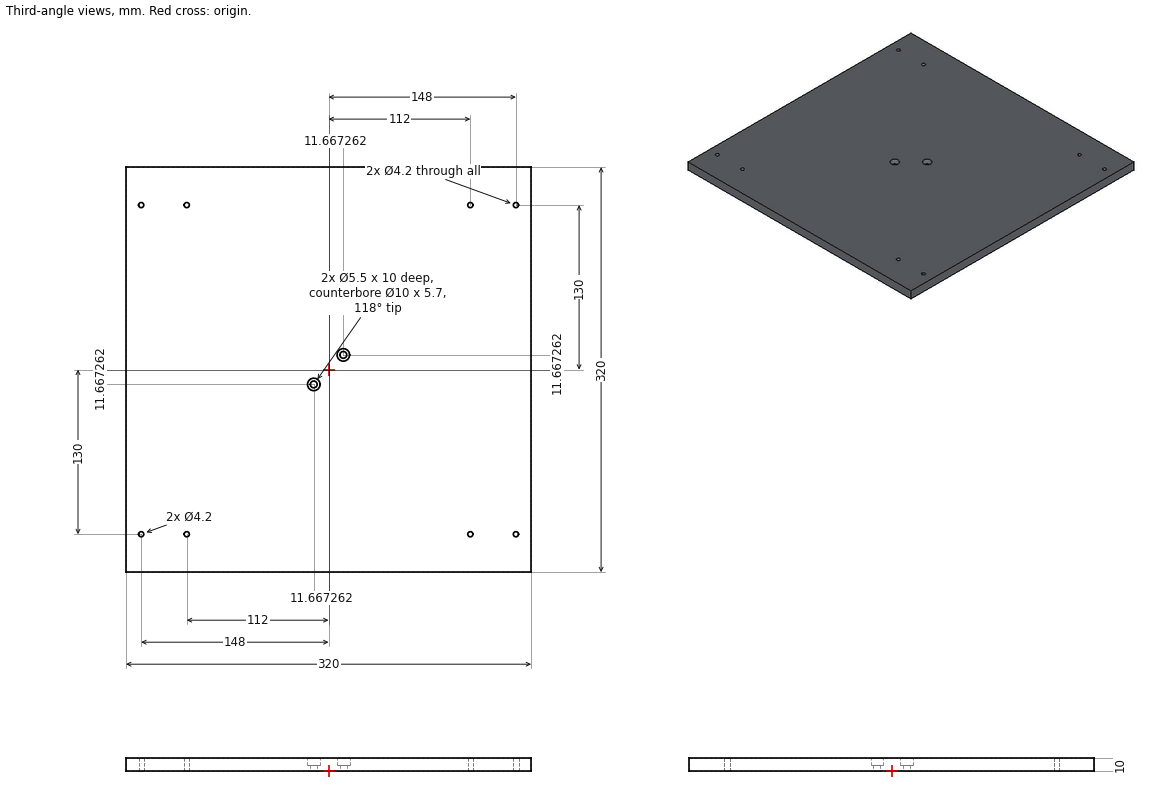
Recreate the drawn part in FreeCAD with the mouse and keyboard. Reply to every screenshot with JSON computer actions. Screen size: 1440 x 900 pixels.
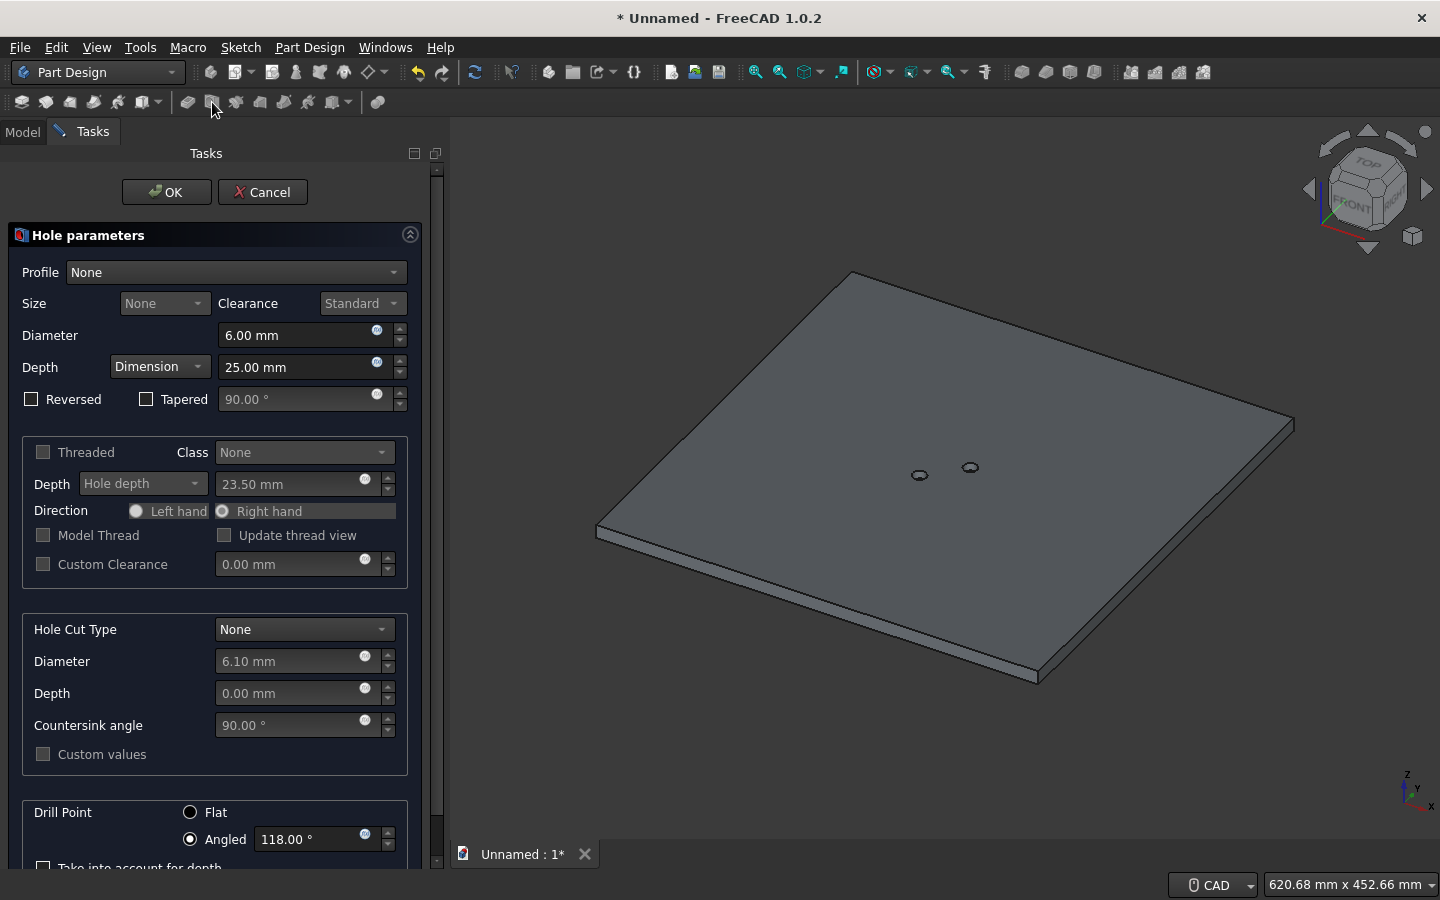
{"action": "triple_click", "coordinate": [305, 335]}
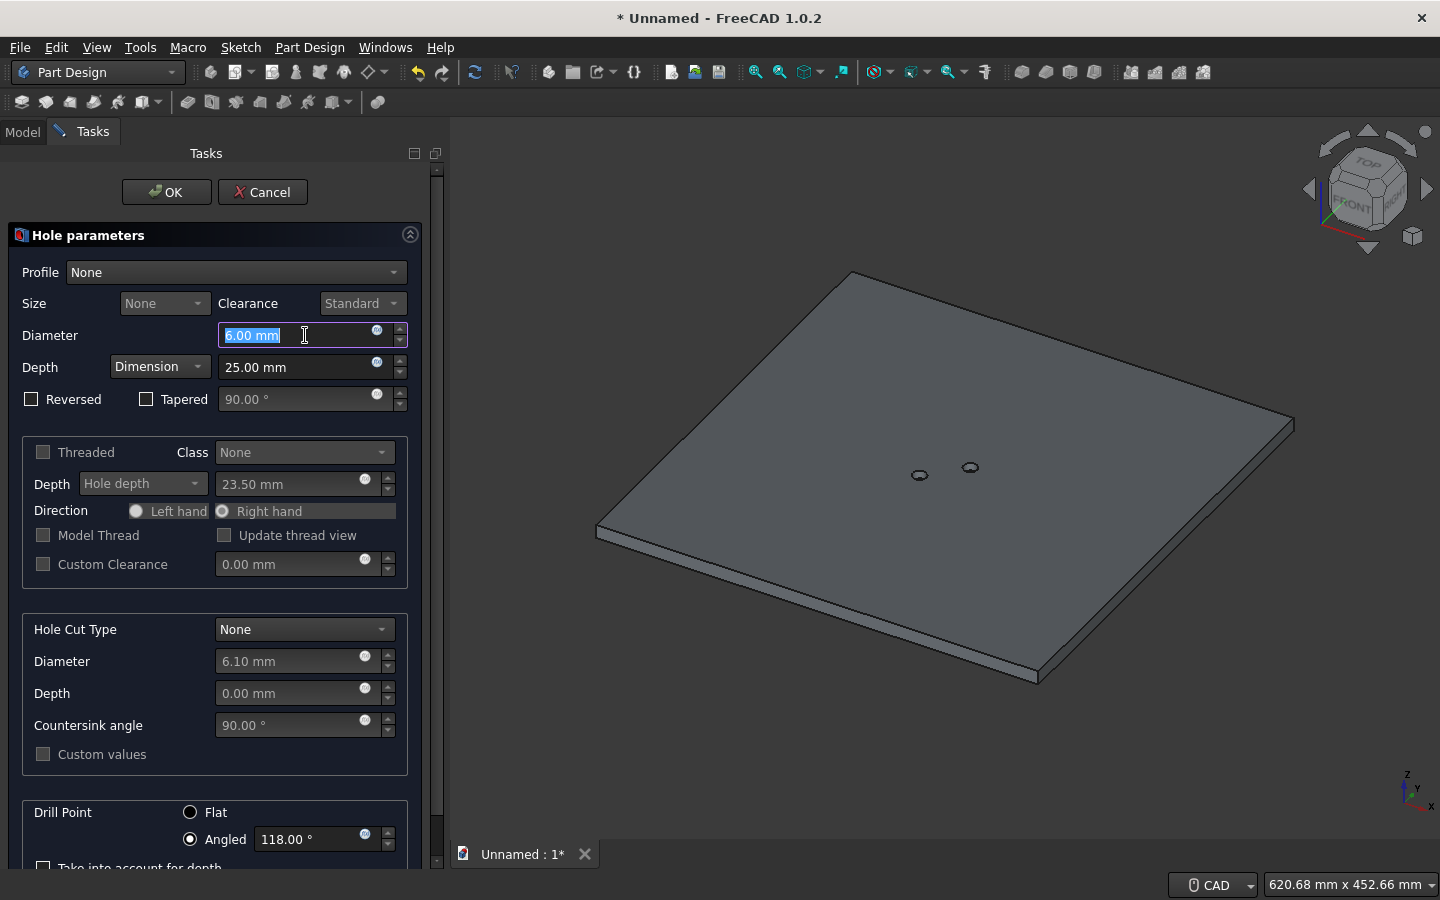
{"action": "type", "text": "4.2"}
{"action": "key", "text": "Tab"}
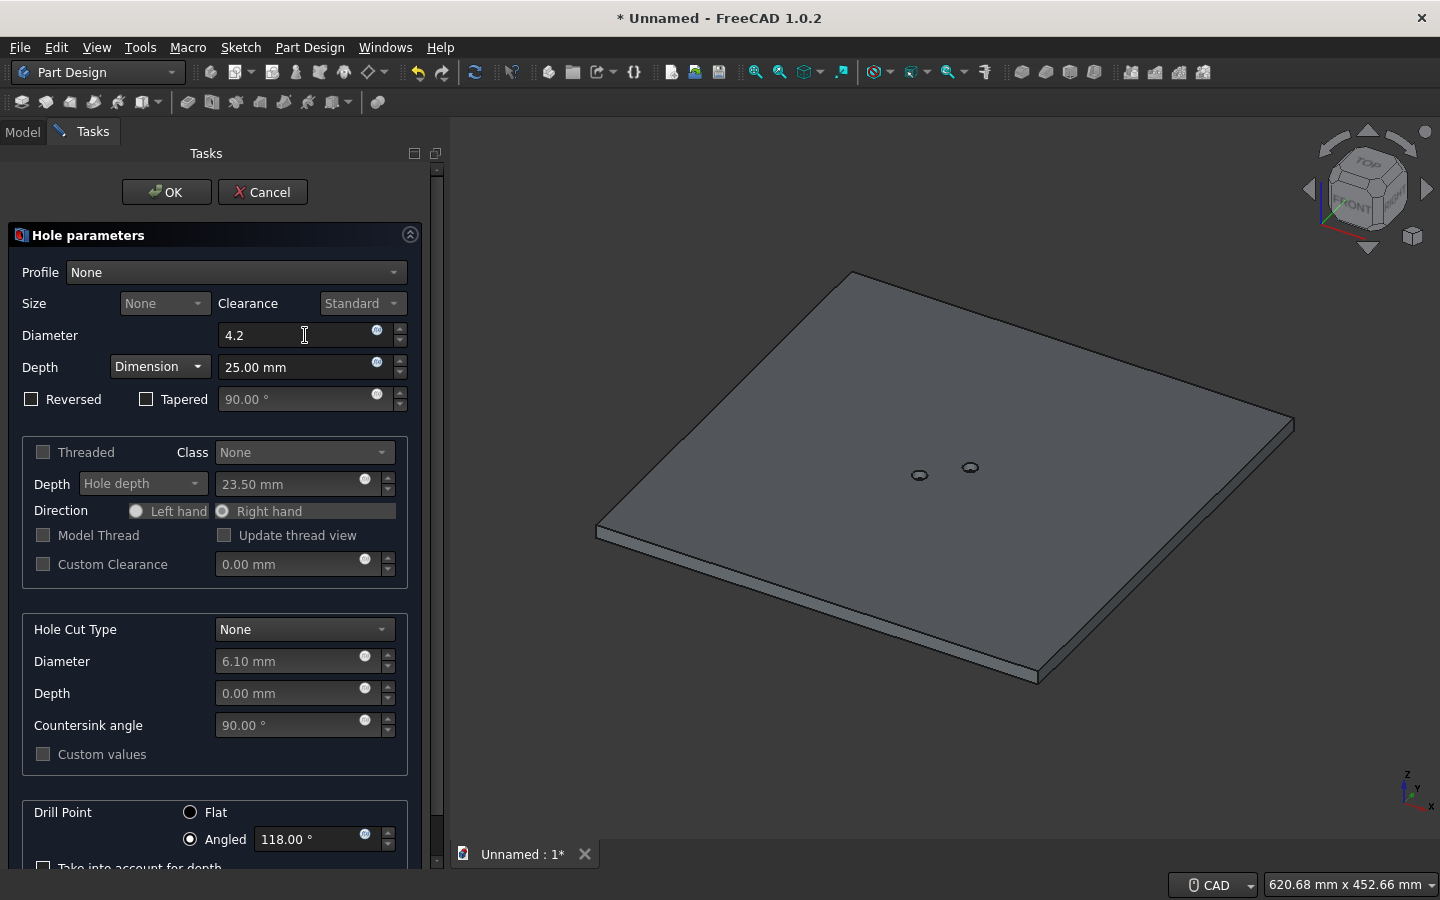
{"action": "left_click", "coordinate": [161, 366]}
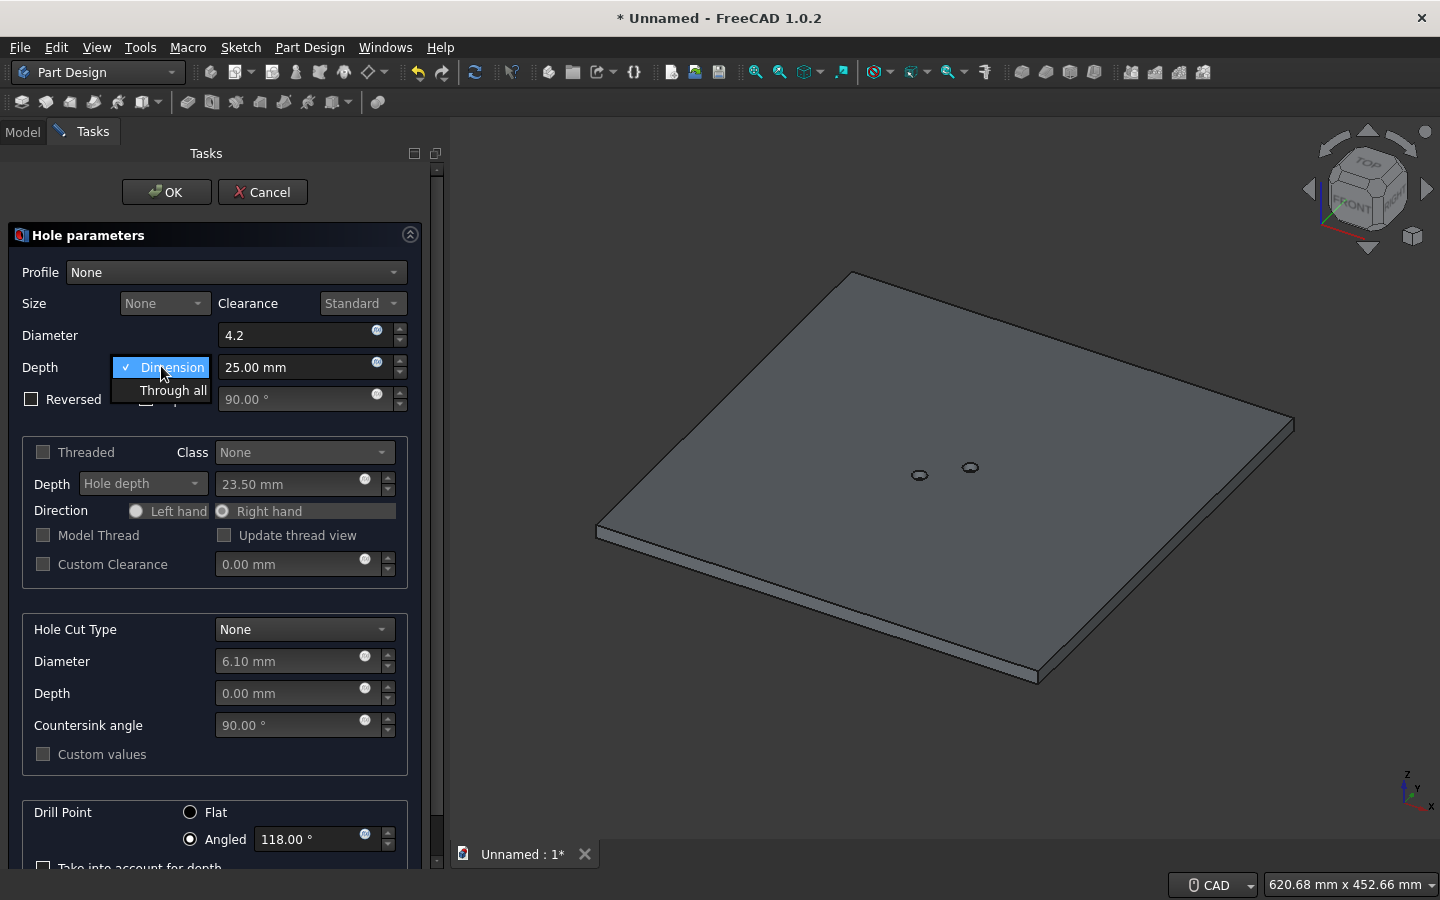
{"action": "left_click", "coordinate": [160, 390]}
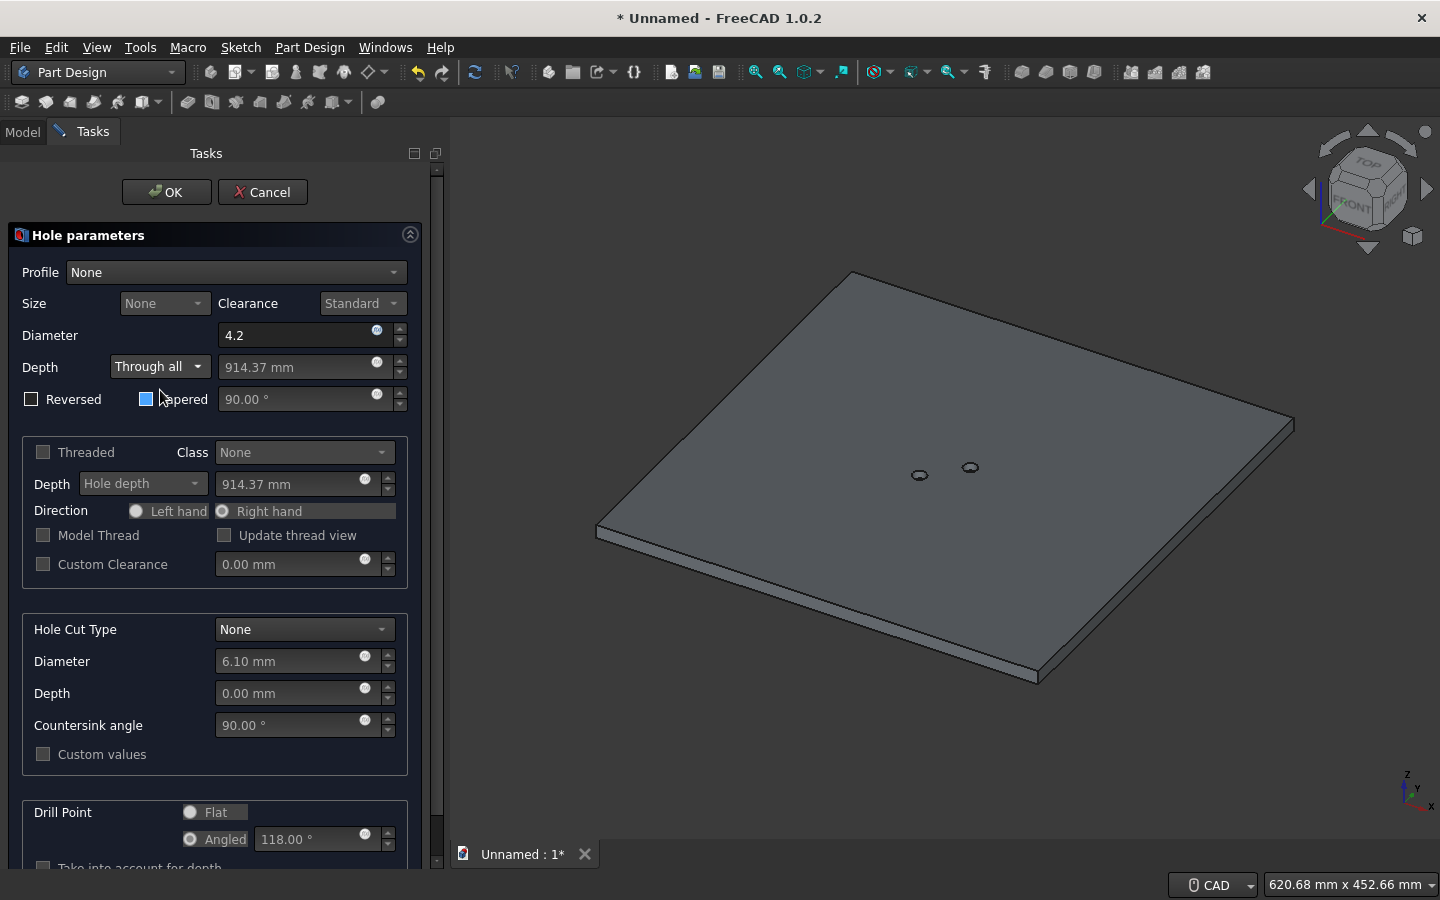
{"action": "left_click", "coordinate": [30, 399]}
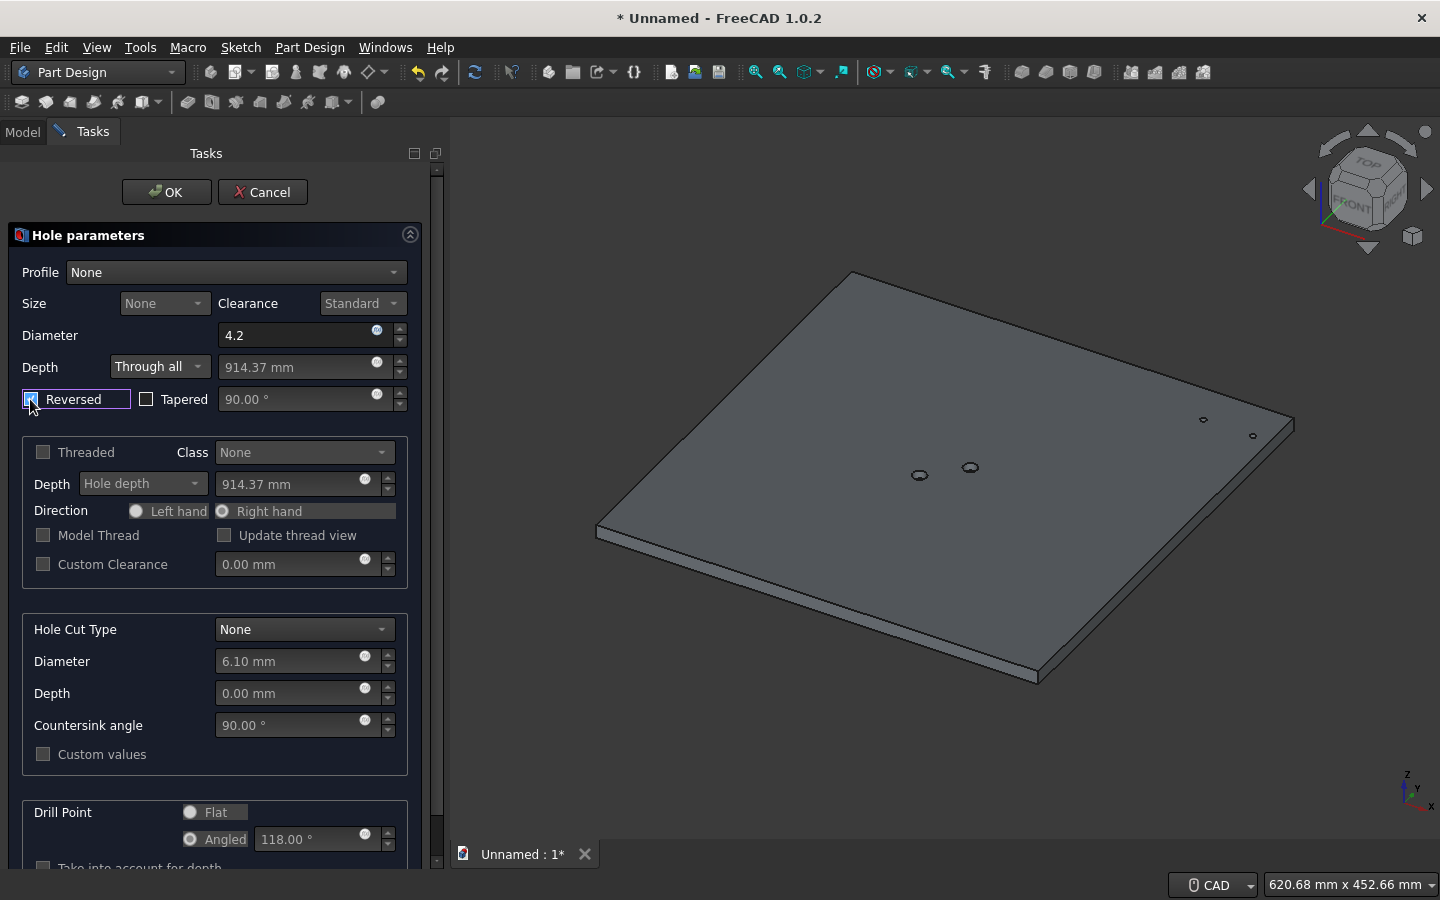
{"action": "left_click", "coordinate": [167, 192]}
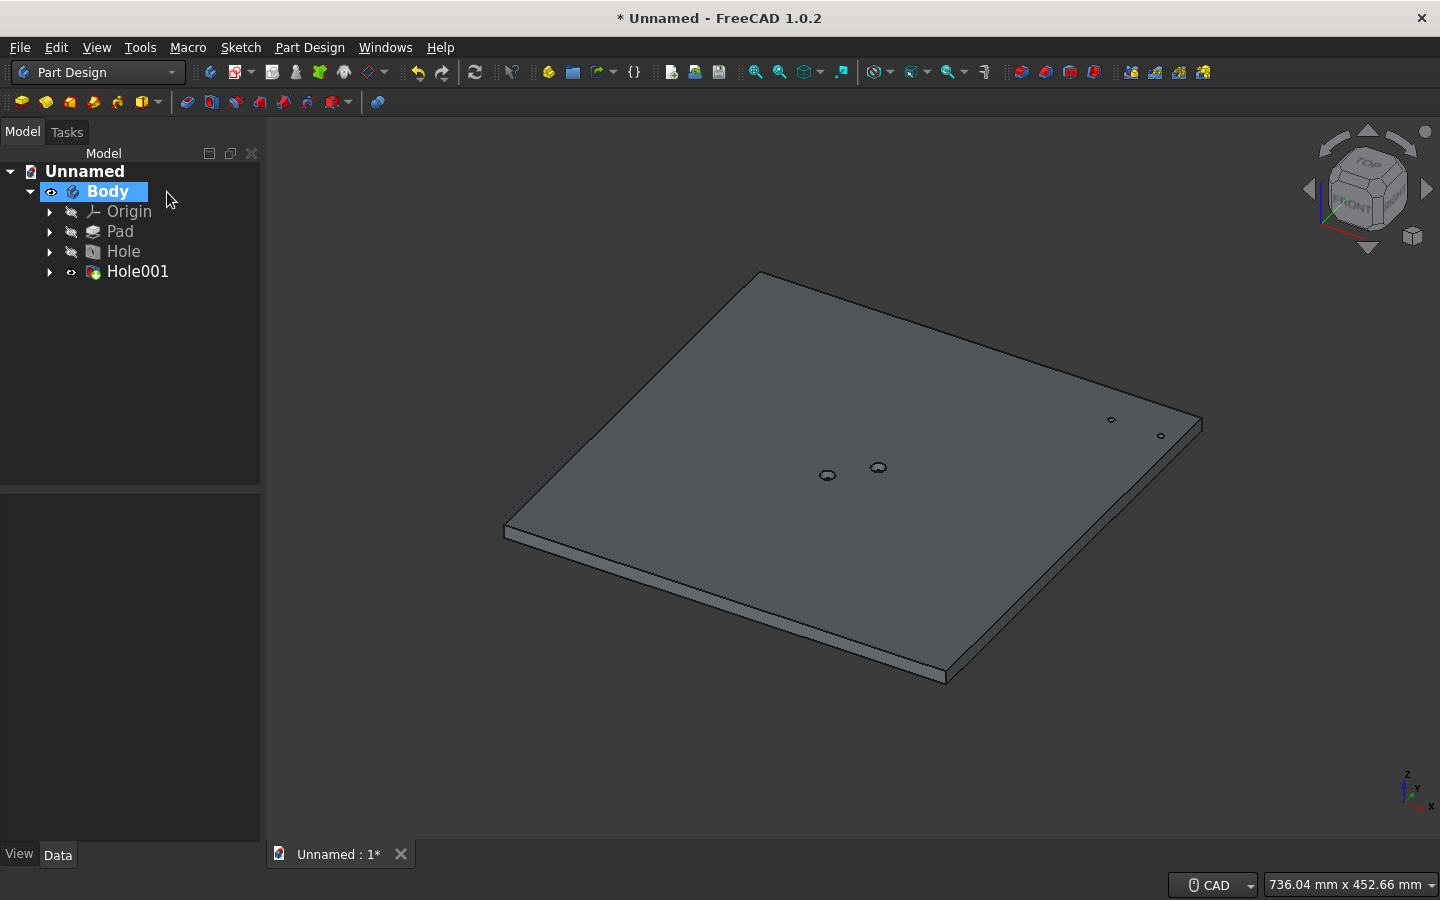
{"action": "left_click", "coordinate": [116, 272]}